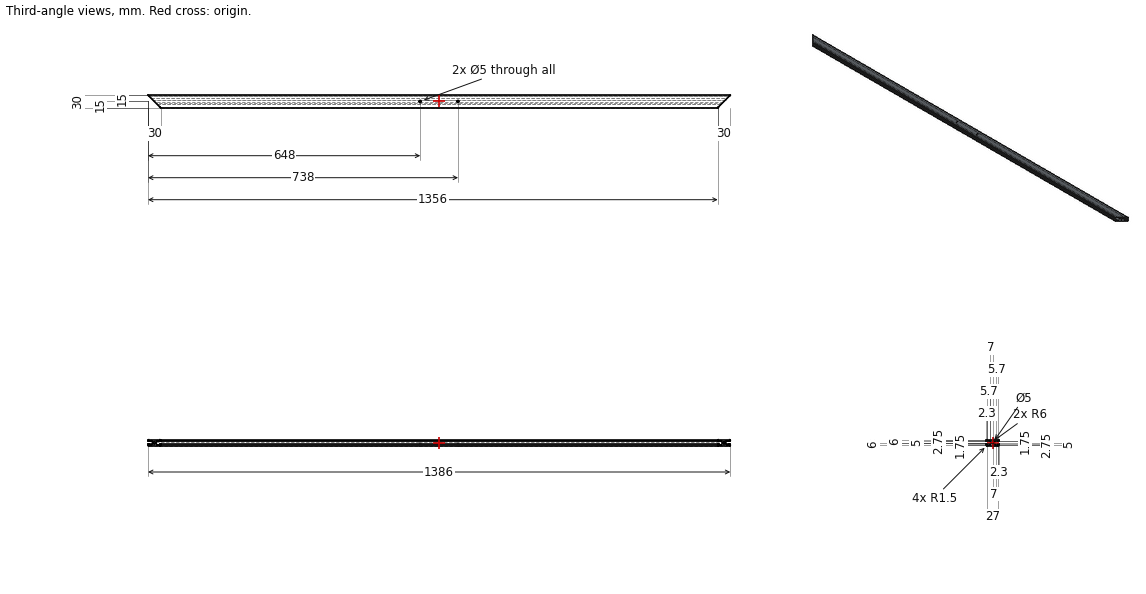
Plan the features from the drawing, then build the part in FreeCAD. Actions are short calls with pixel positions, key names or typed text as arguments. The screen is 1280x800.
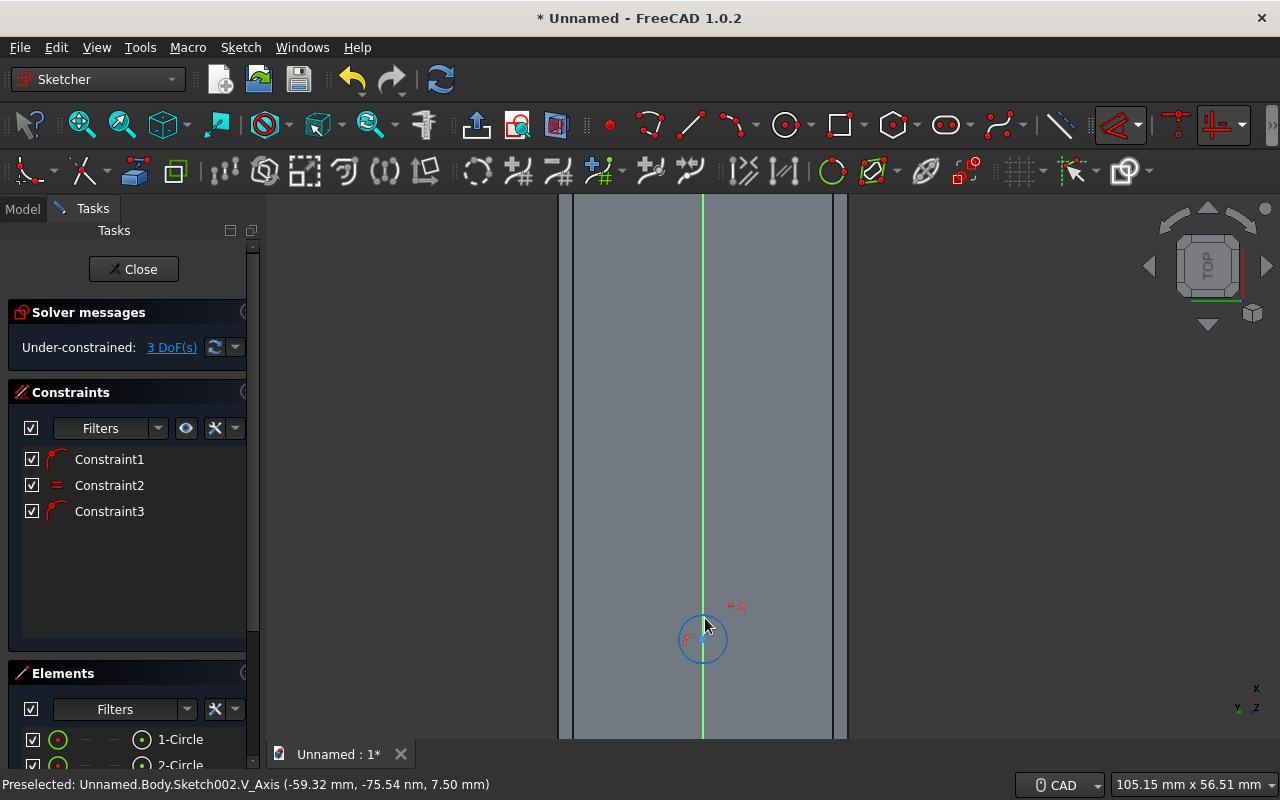
click(704, 615)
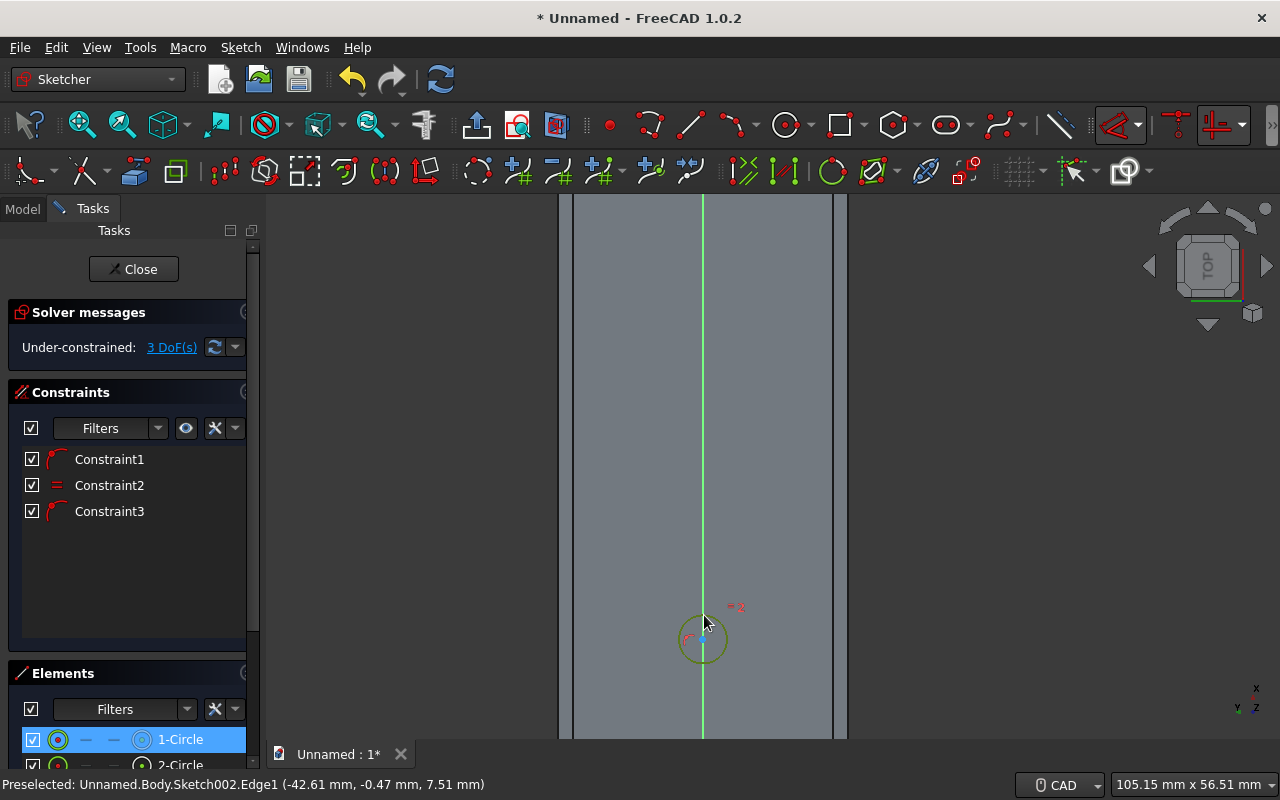
key(k)
key(o)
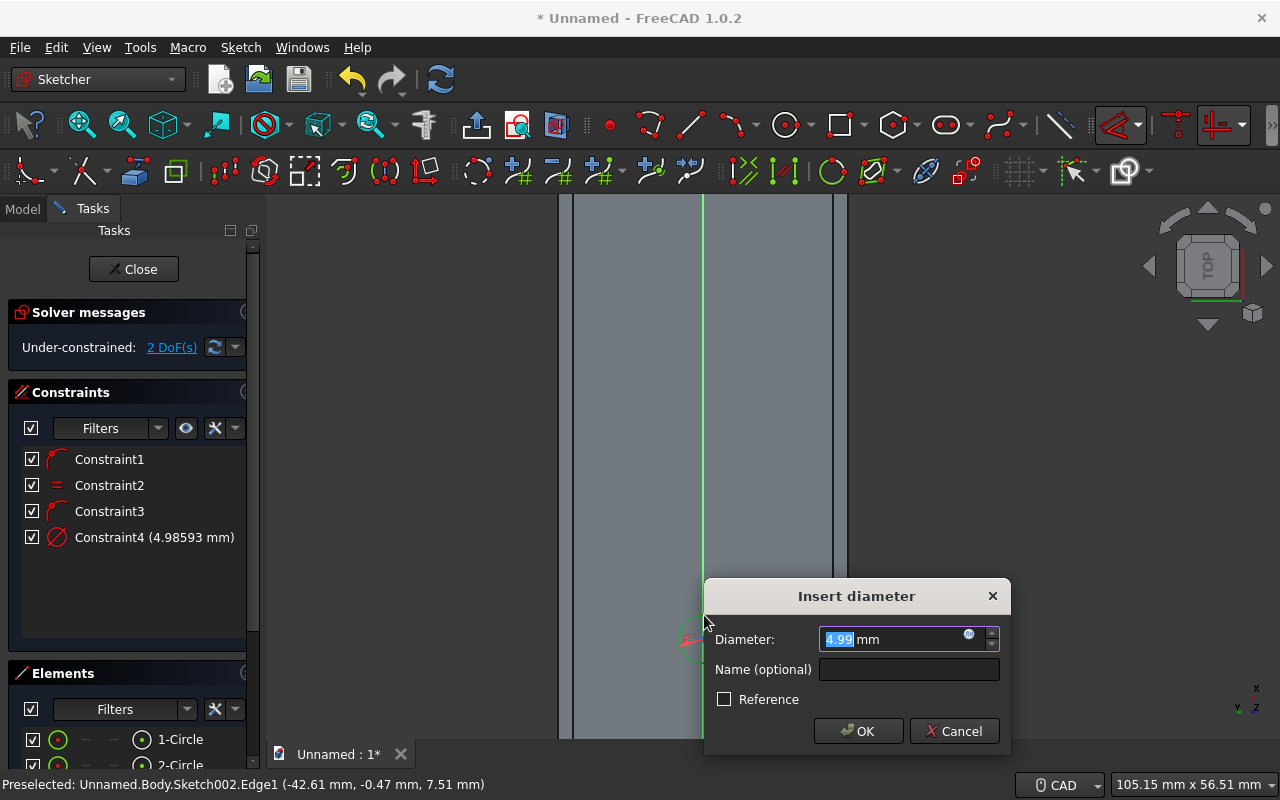
text(5)
key(Return)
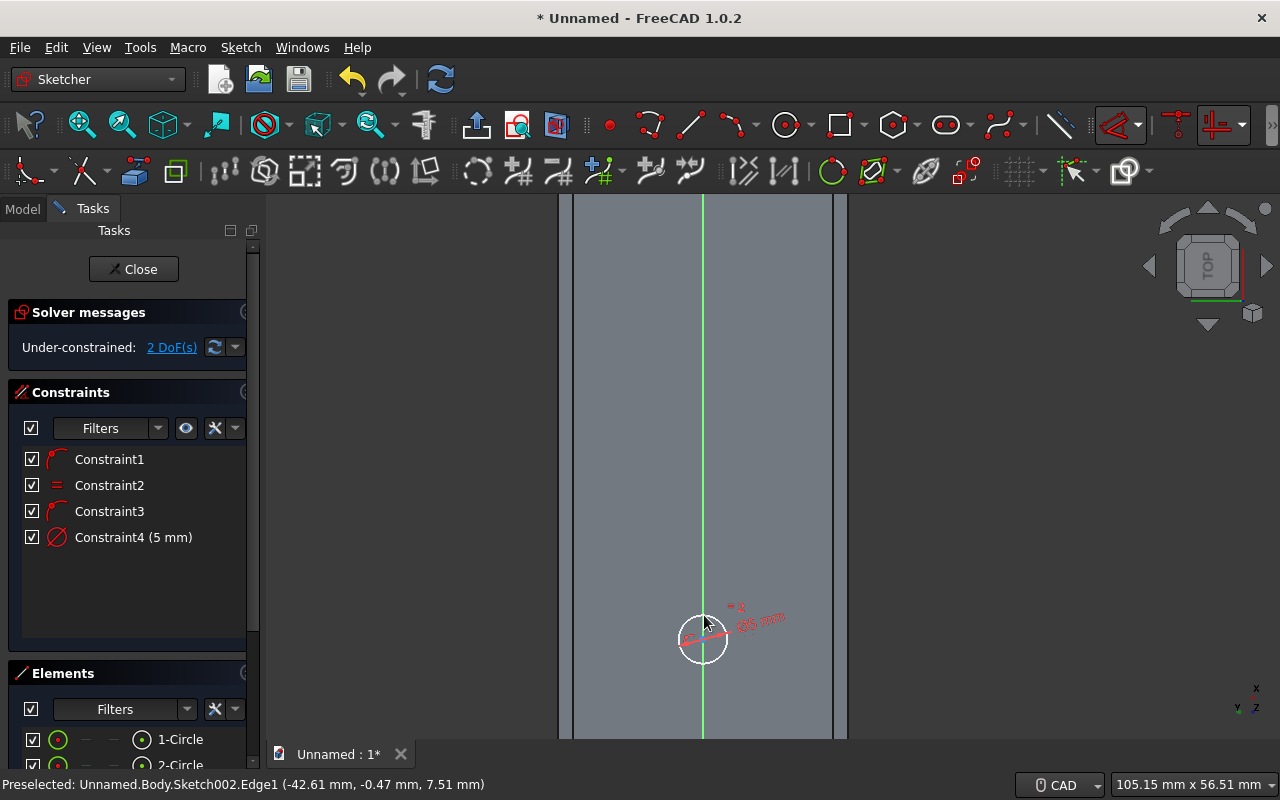
click(703, 639)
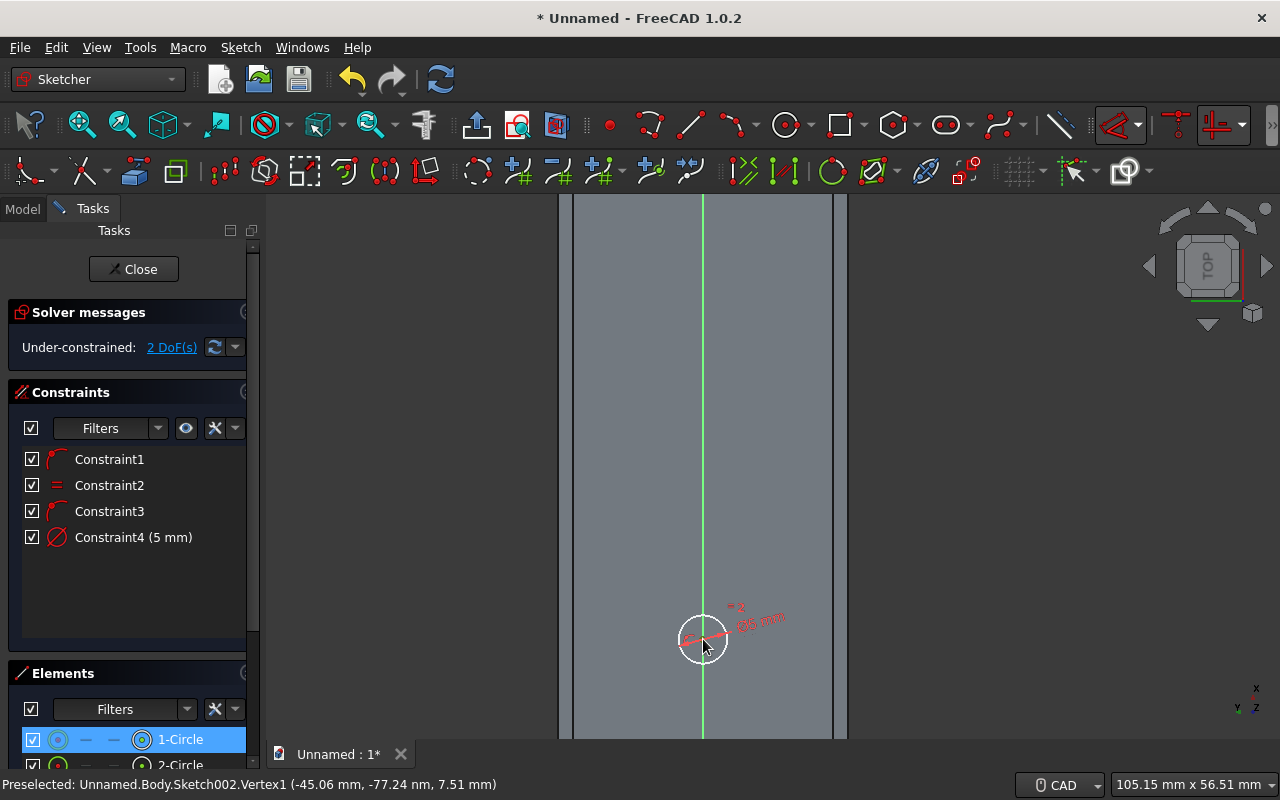
key(i)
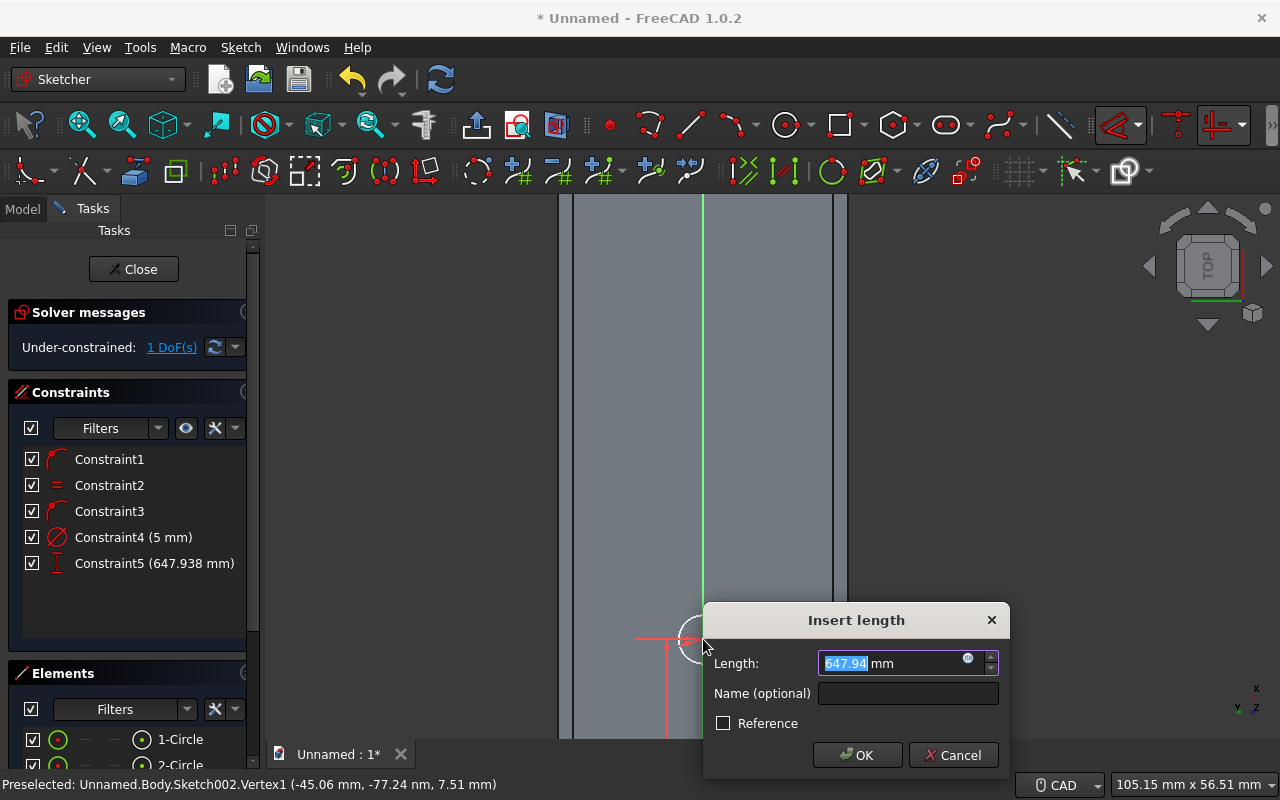
text(648)
key(Return)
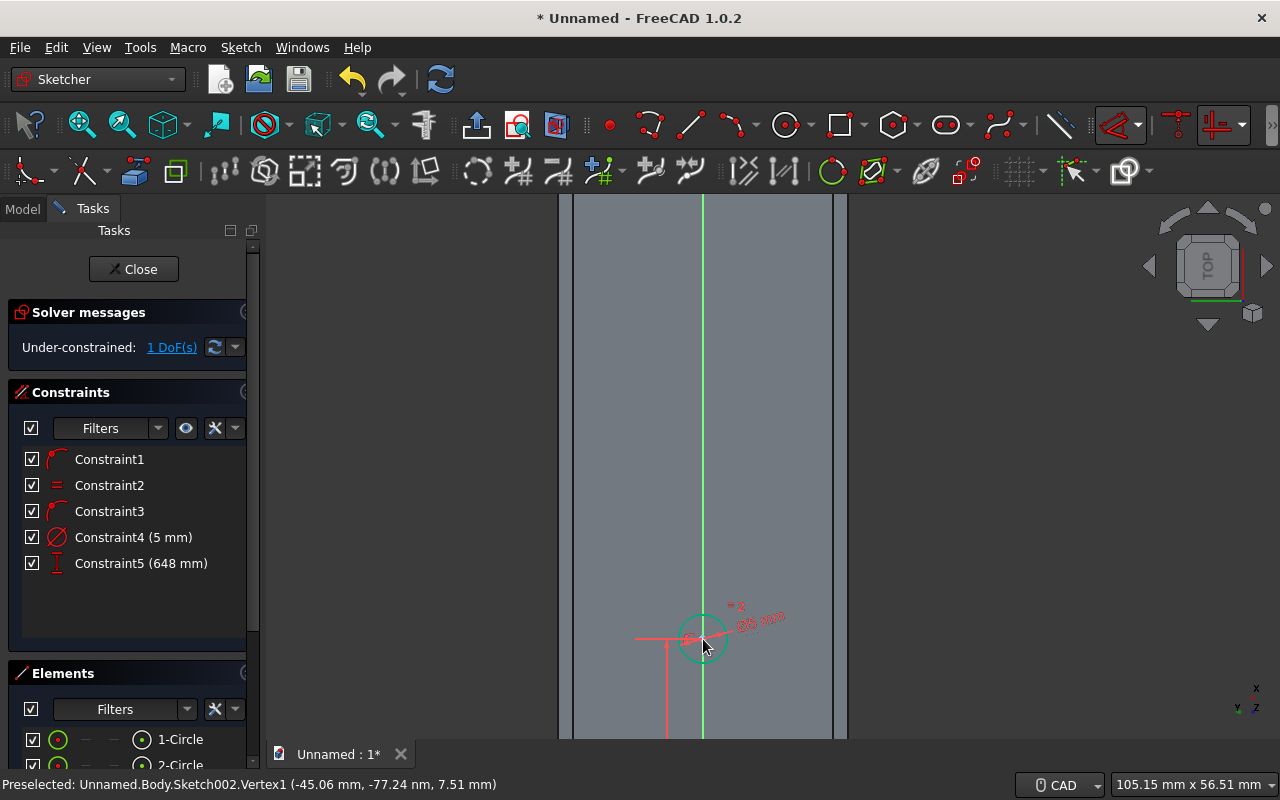
scroll(705, 619, down, 5)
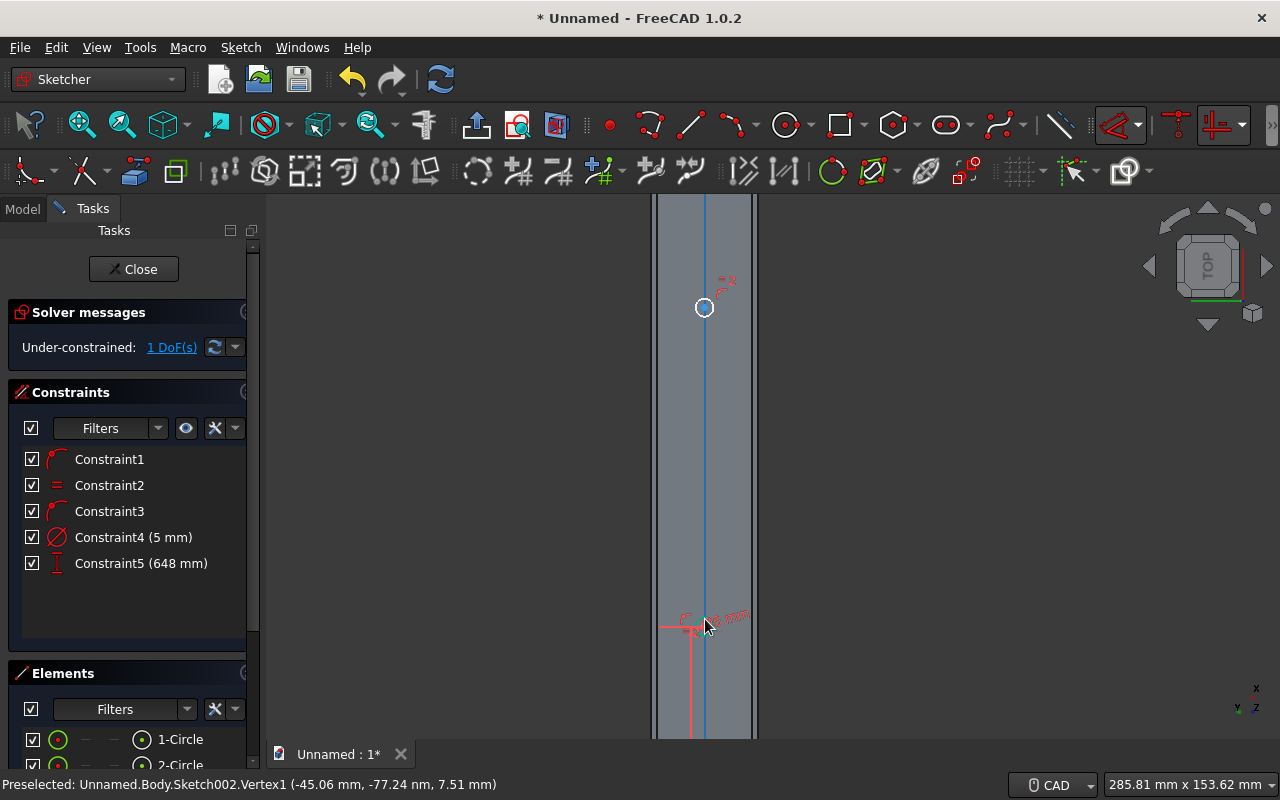
click(705, 308)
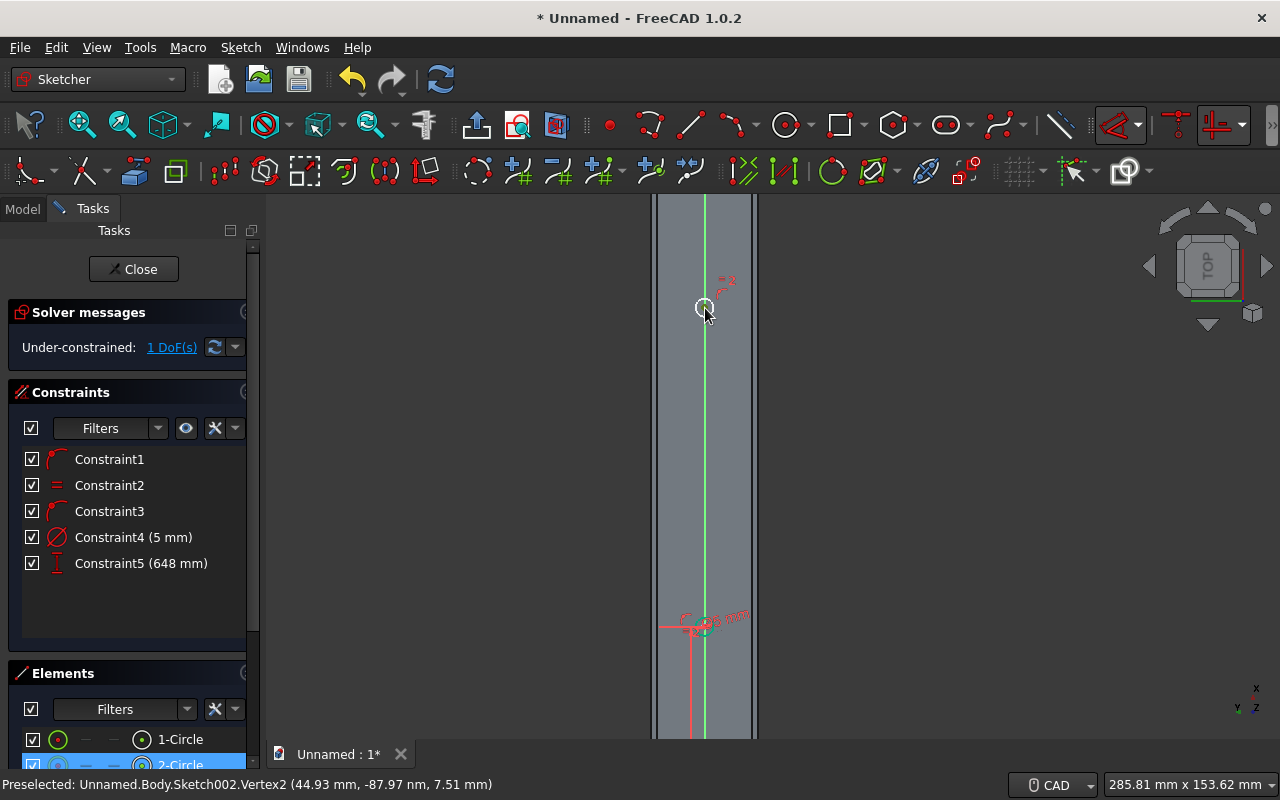
click(1140, 126)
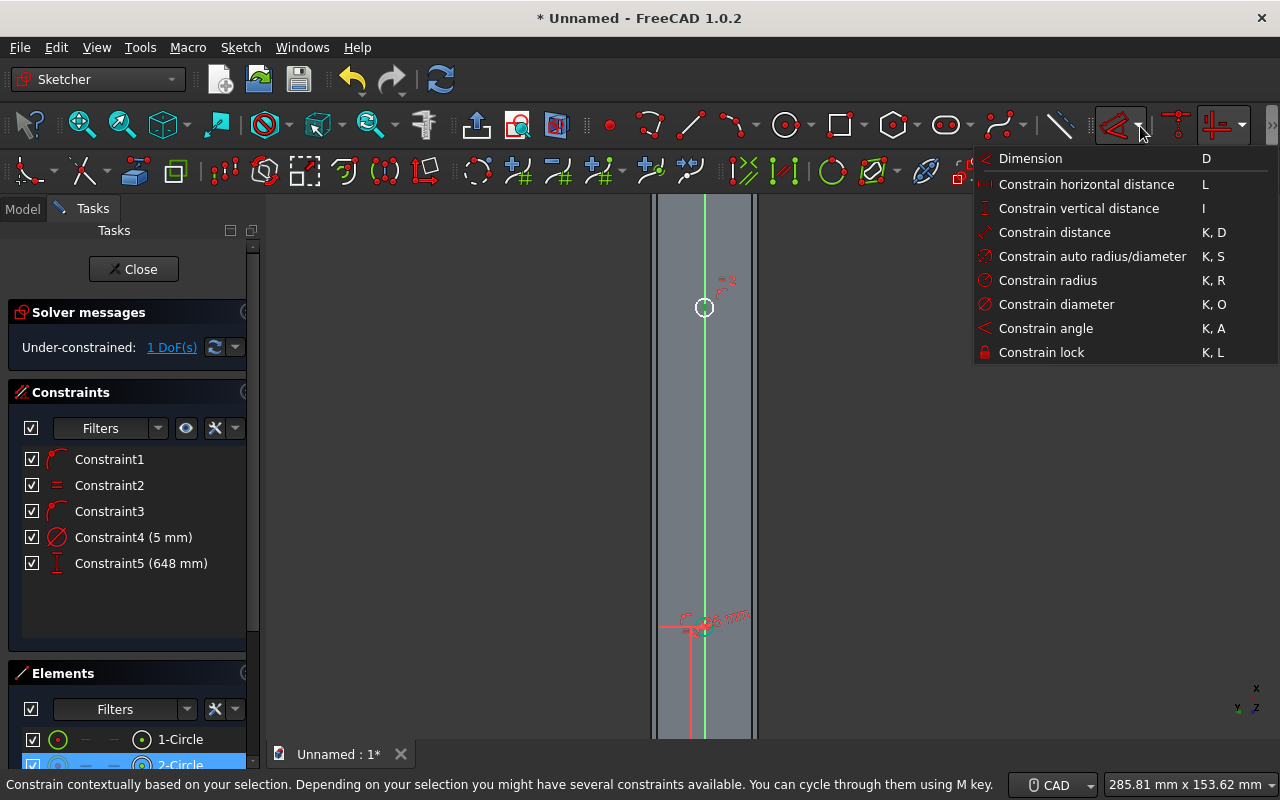
click(1126, 208)